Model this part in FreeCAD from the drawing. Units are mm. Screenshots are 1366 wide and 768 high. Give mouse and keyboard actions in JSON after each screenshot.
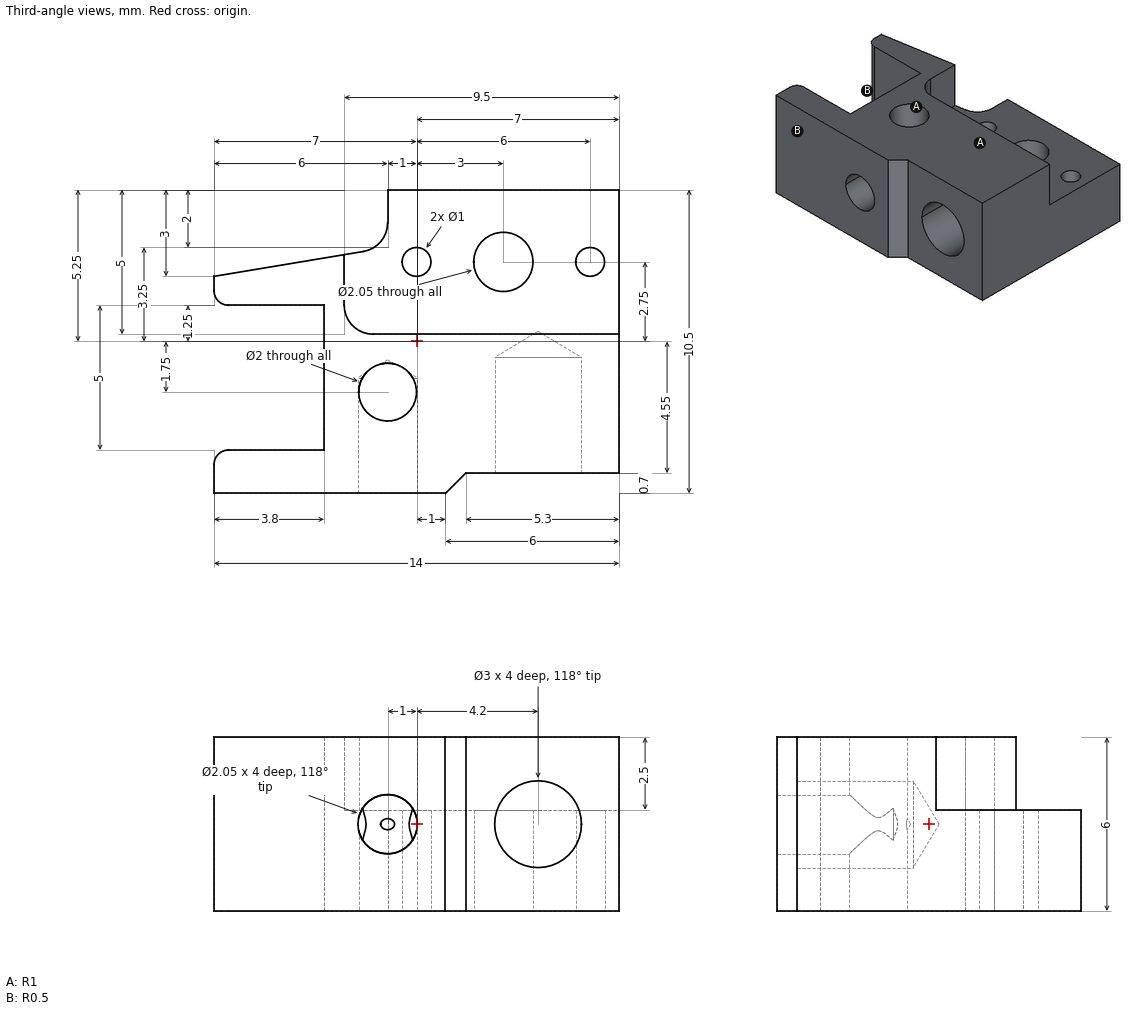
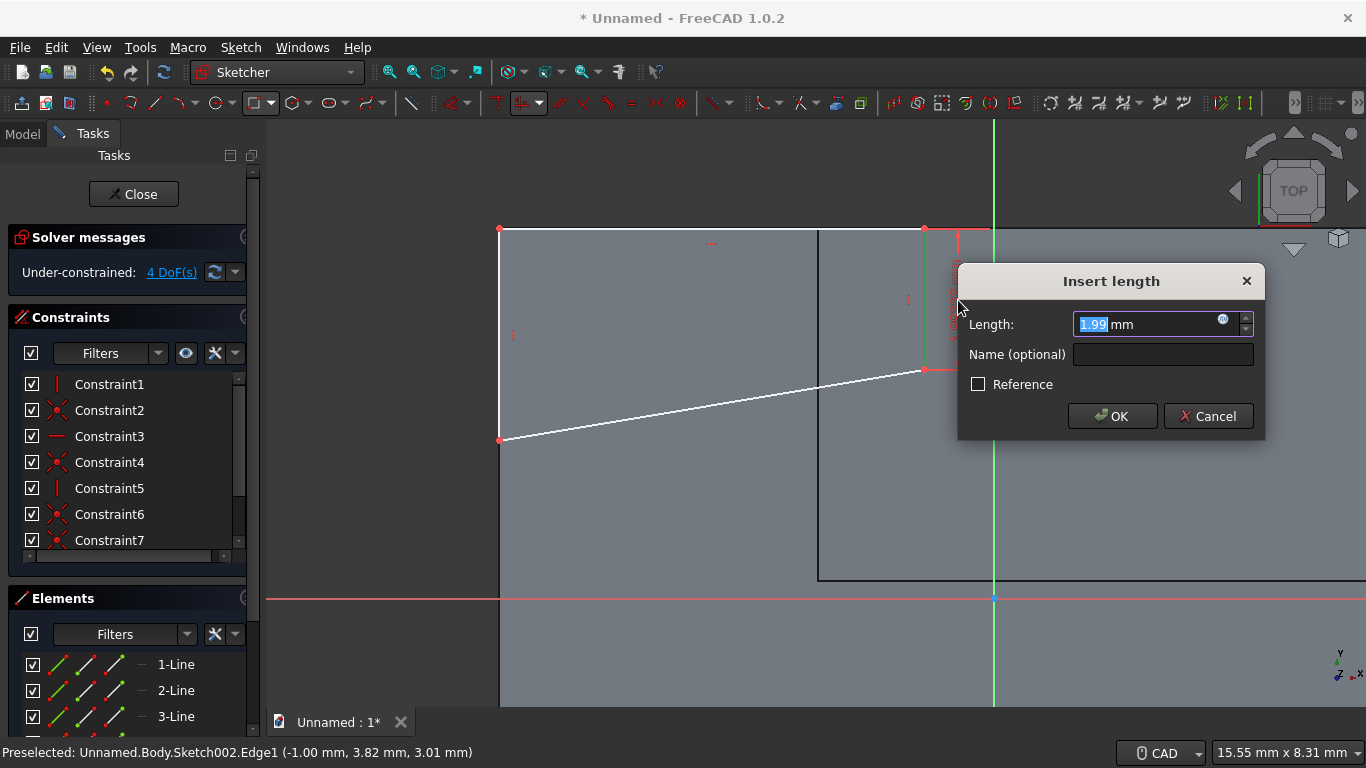
{"action": "type", "text": "2"}
{"action": "key", "text": "Return"}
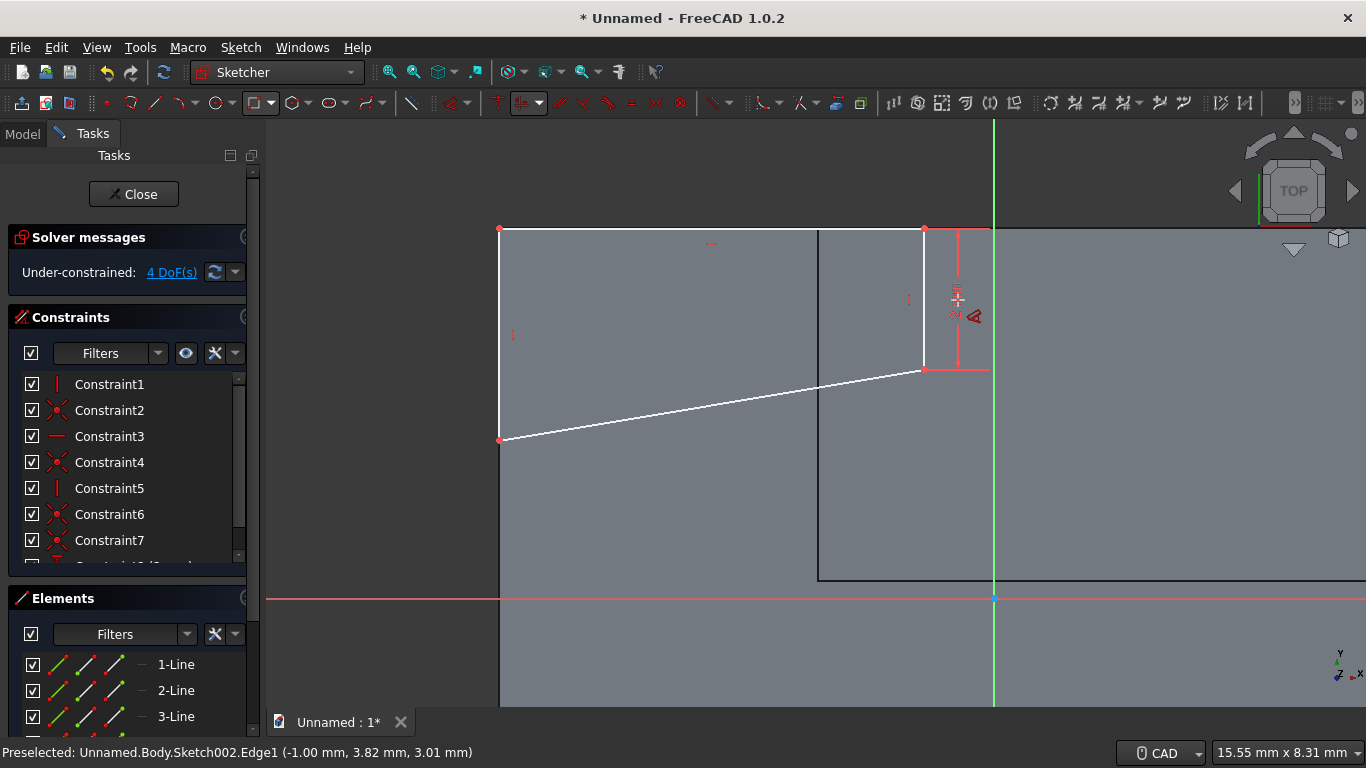
{"action": "left_click", "coordinate": [797, 229]}
{"action": "left_click", "coordinate": [712, 195]}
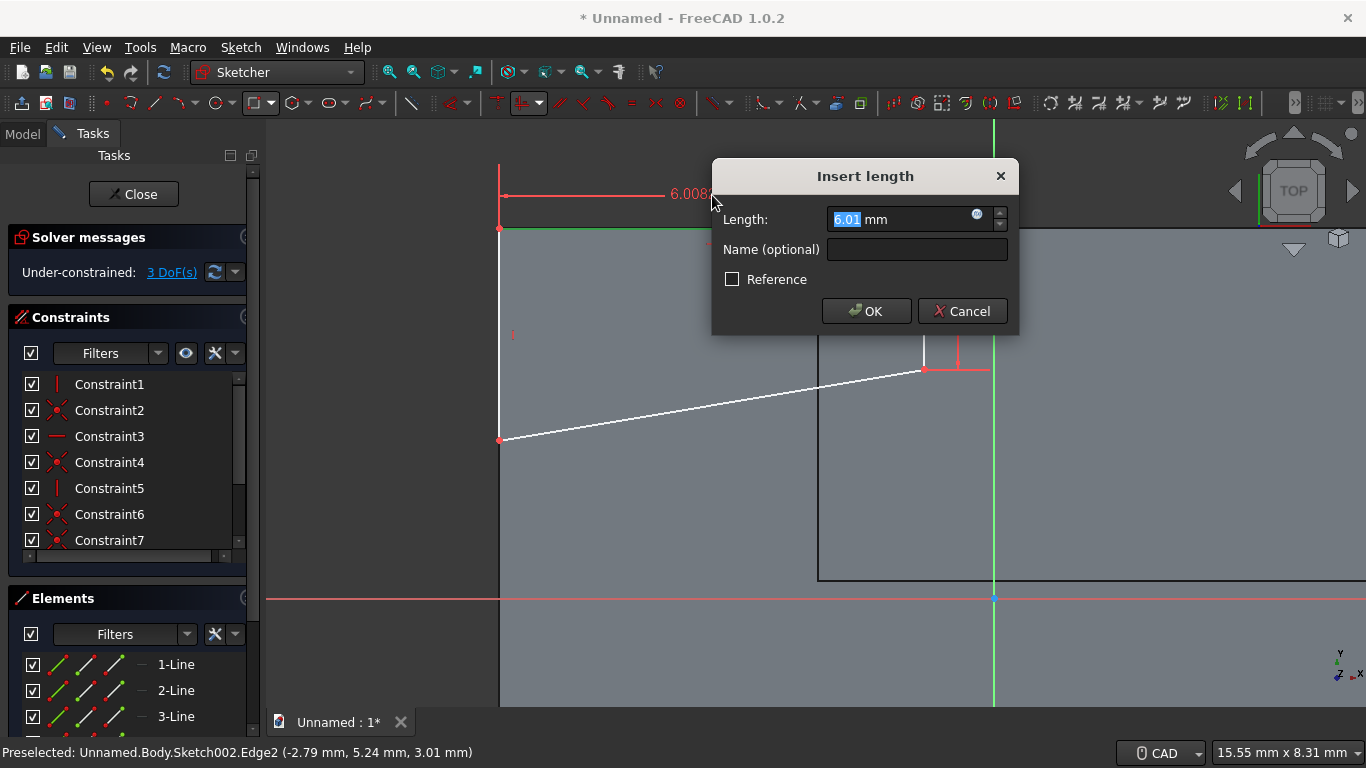
{"action": "type", "text": "6"}
{"action": "key", "text": "Return"}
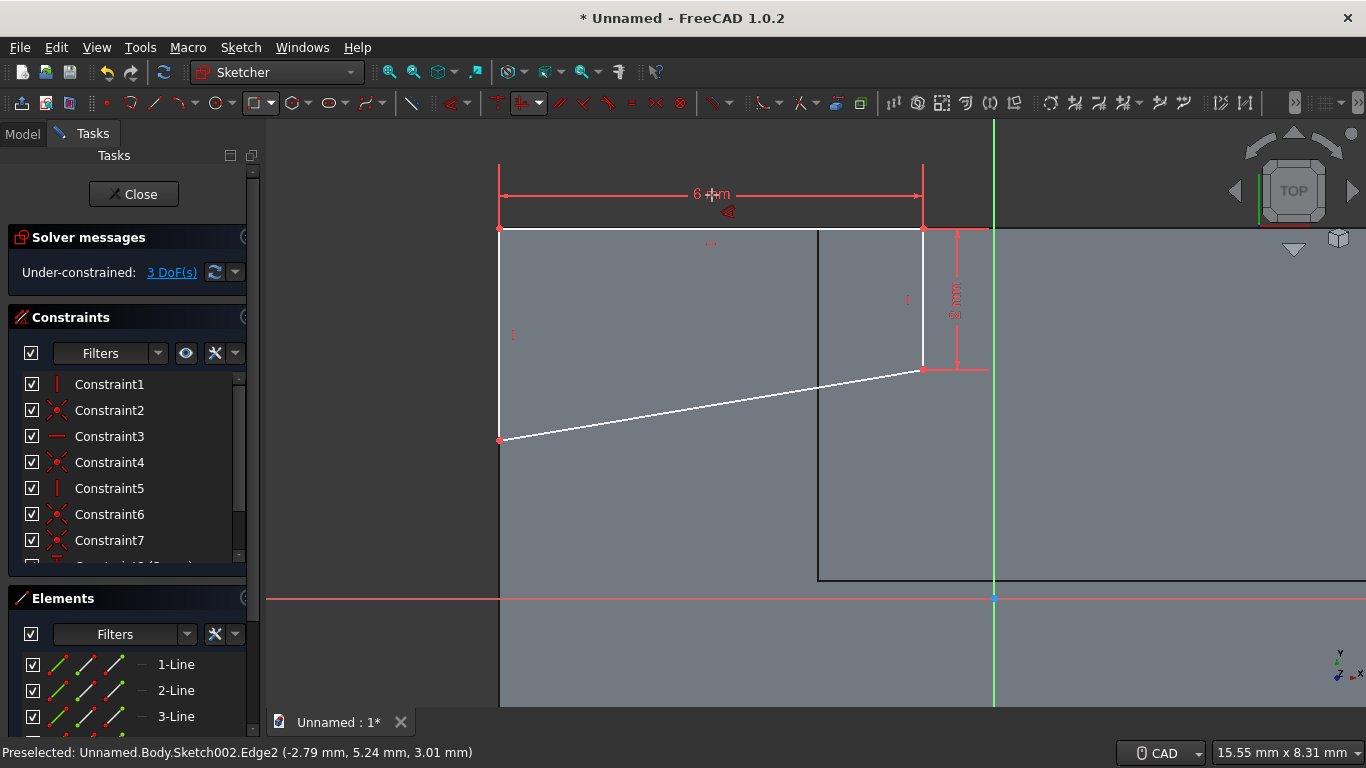
{"action": "left_click", "coordinate": [499, 292]}
{"action": "left_click", "coordinate": [465, 335]}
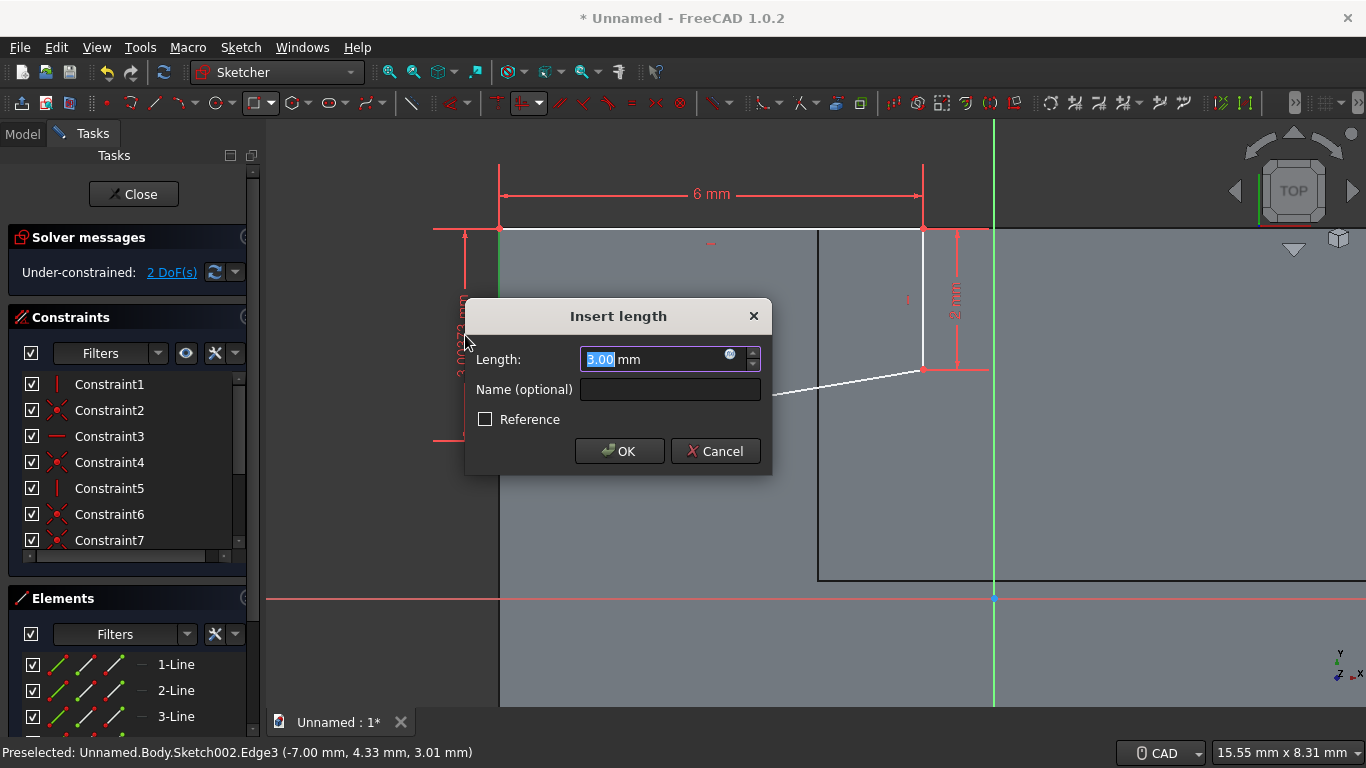
{"action": "type", "text": "3"}
{"action": "key", "text": "Return"}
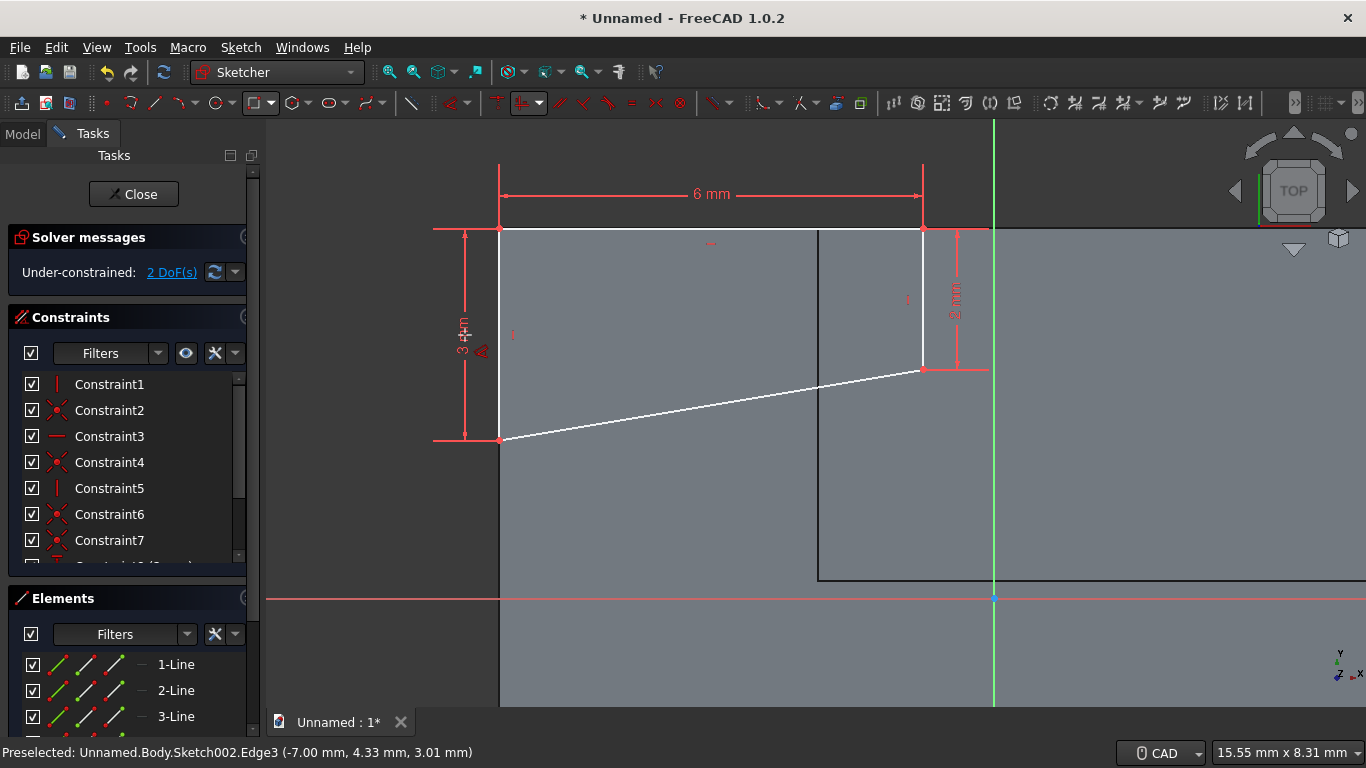
{"action": "left_click", "coordinate": [923, 370]}
{"action": "left_click", "coordinate": [959, 633]}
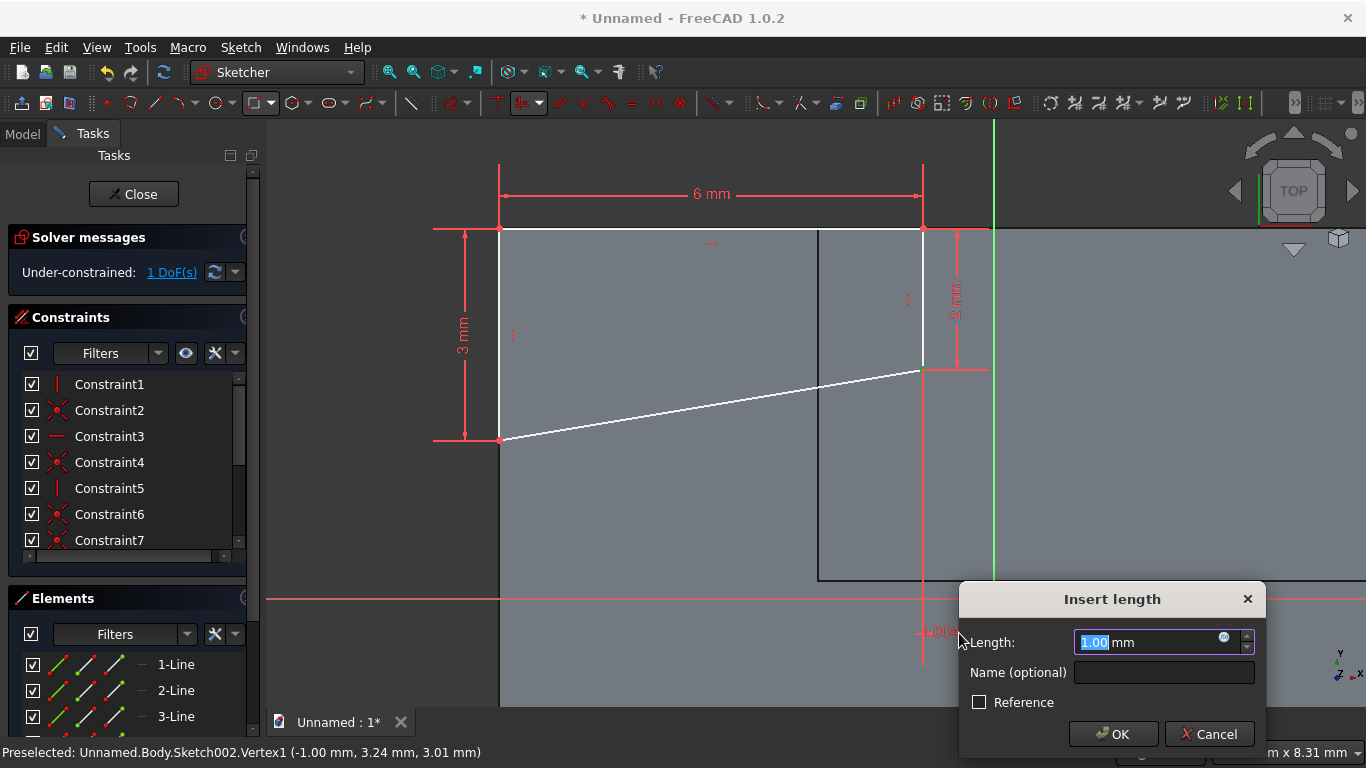
{"action": "type", "text": "1"}
{"action": "key", "text": "Return"}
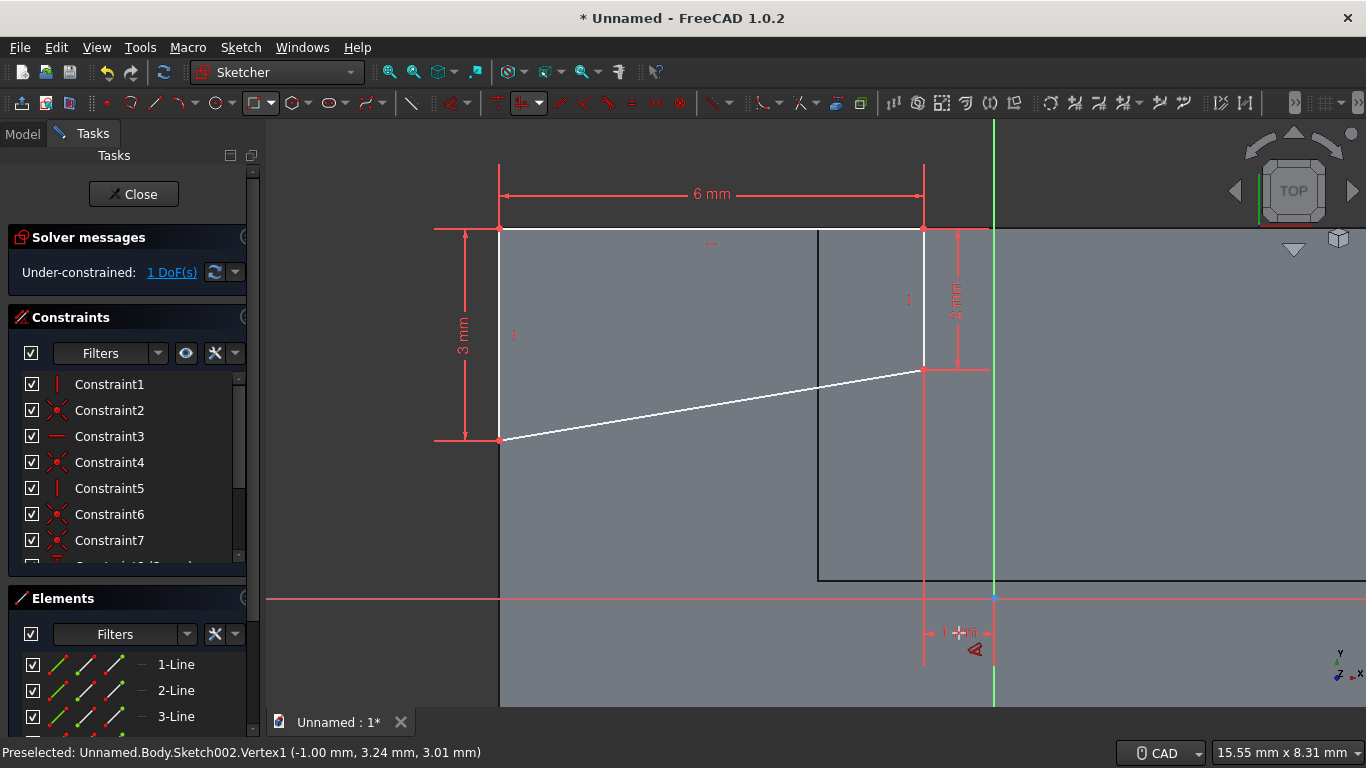
{"action": "left_click", "coordinate": [924, 370]}
{"action": "left_click", "coordinate": [1028, 484]}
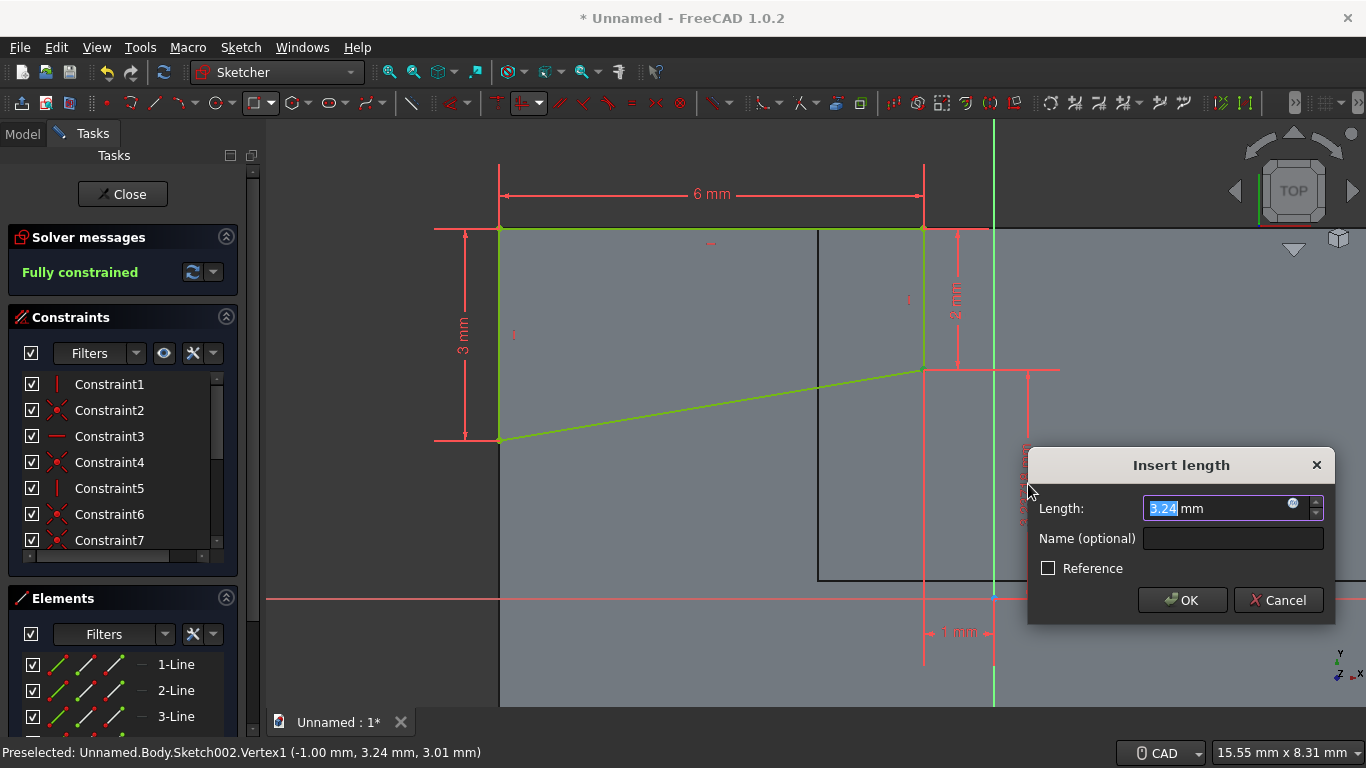
{"action": "type", "text": "3.25"}
{"action": "key", "text": "Return"}
{"action": "key", "text": "Escape"}